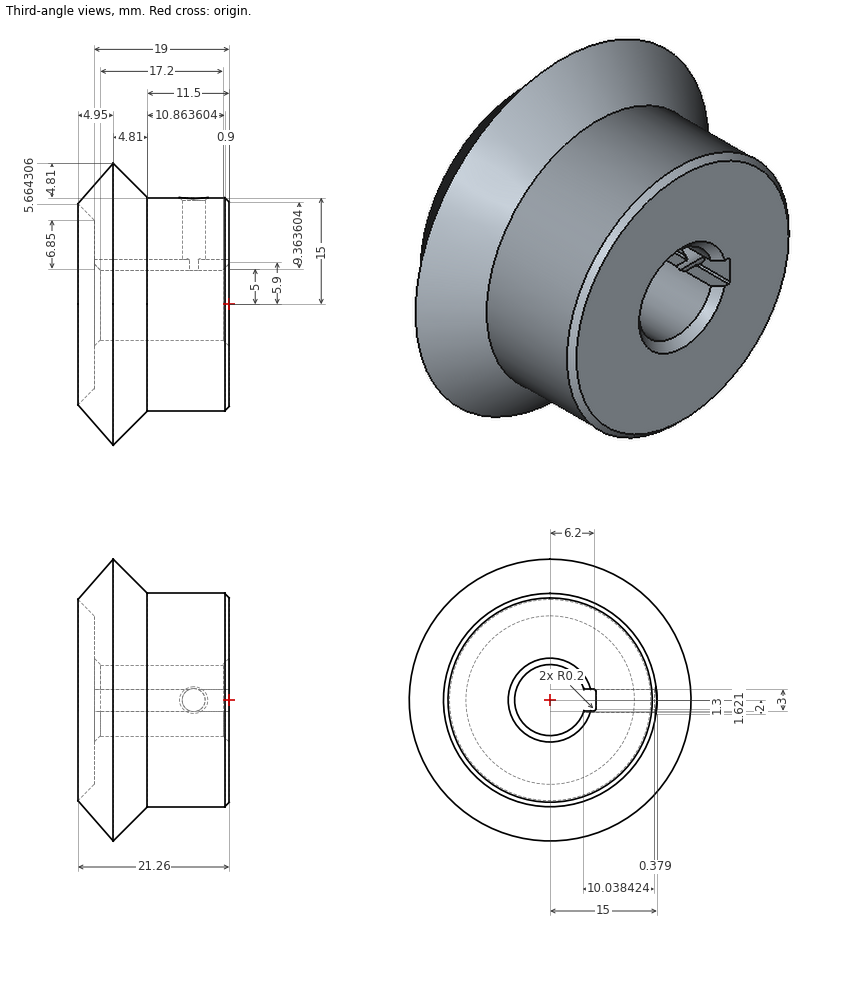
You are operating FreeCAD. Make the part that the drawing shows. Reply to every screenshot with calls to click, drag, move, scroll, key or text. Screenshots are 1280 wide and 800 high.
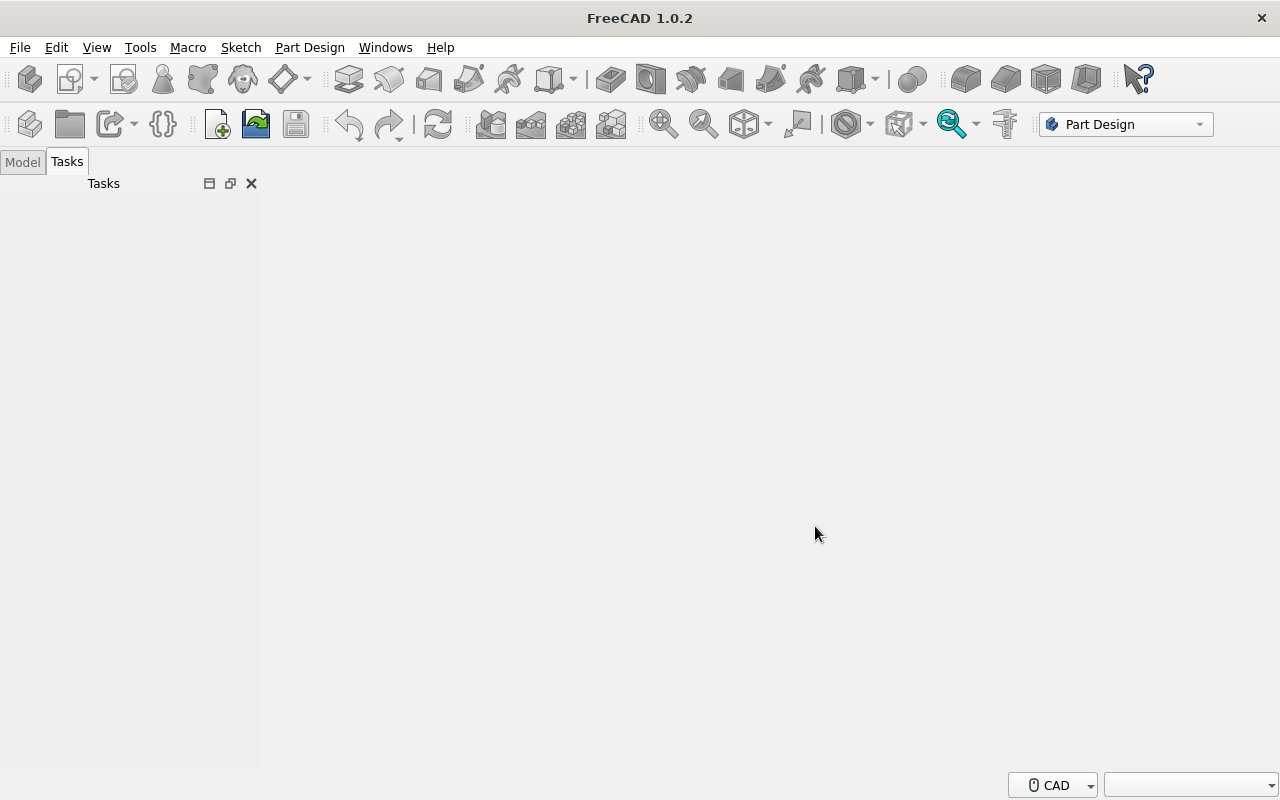
key(ctrl+n)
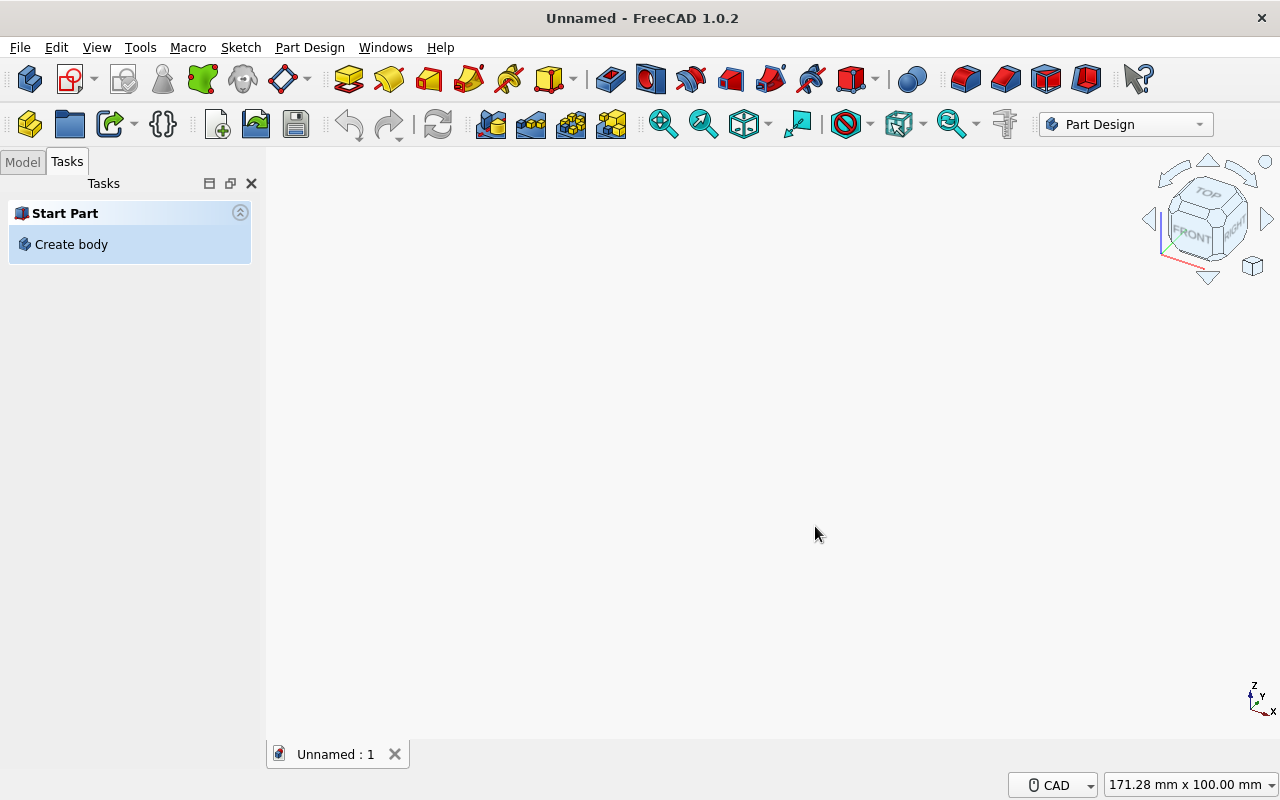
click(70, 80)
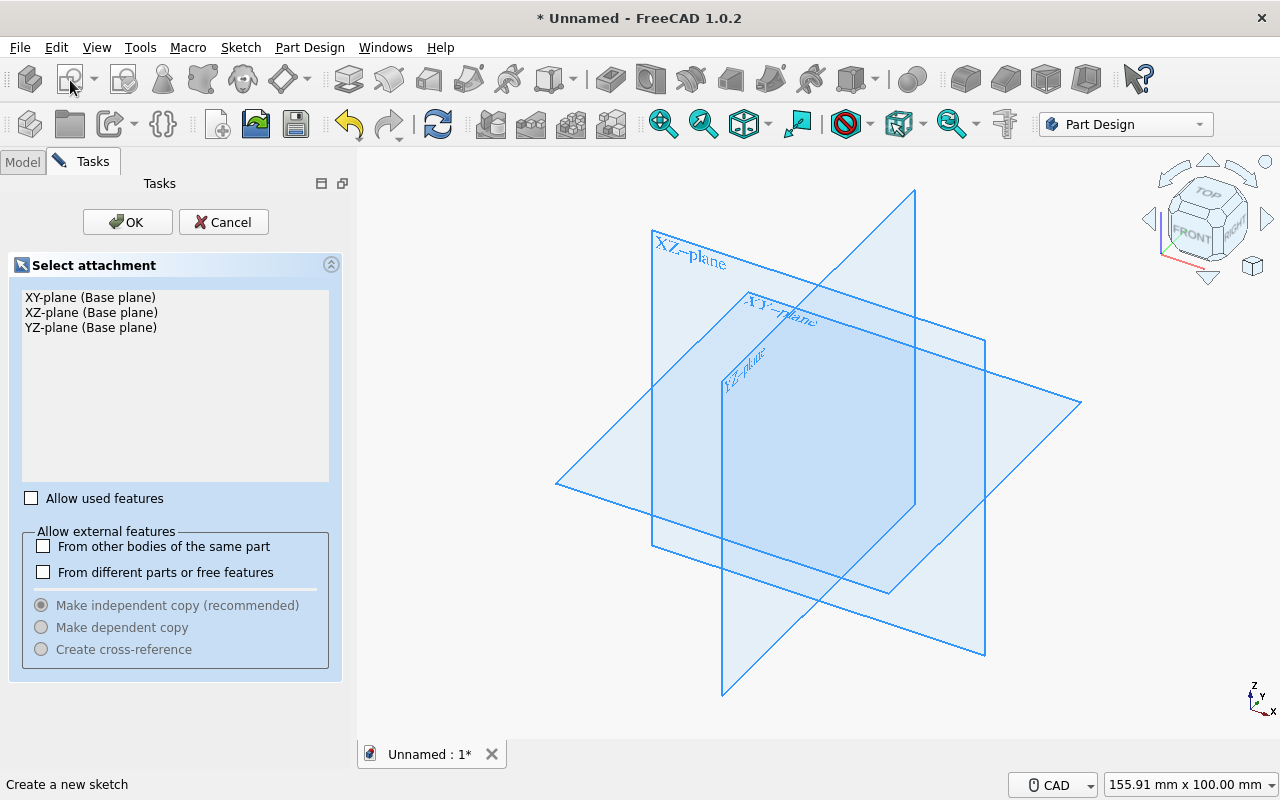
click(82, 298)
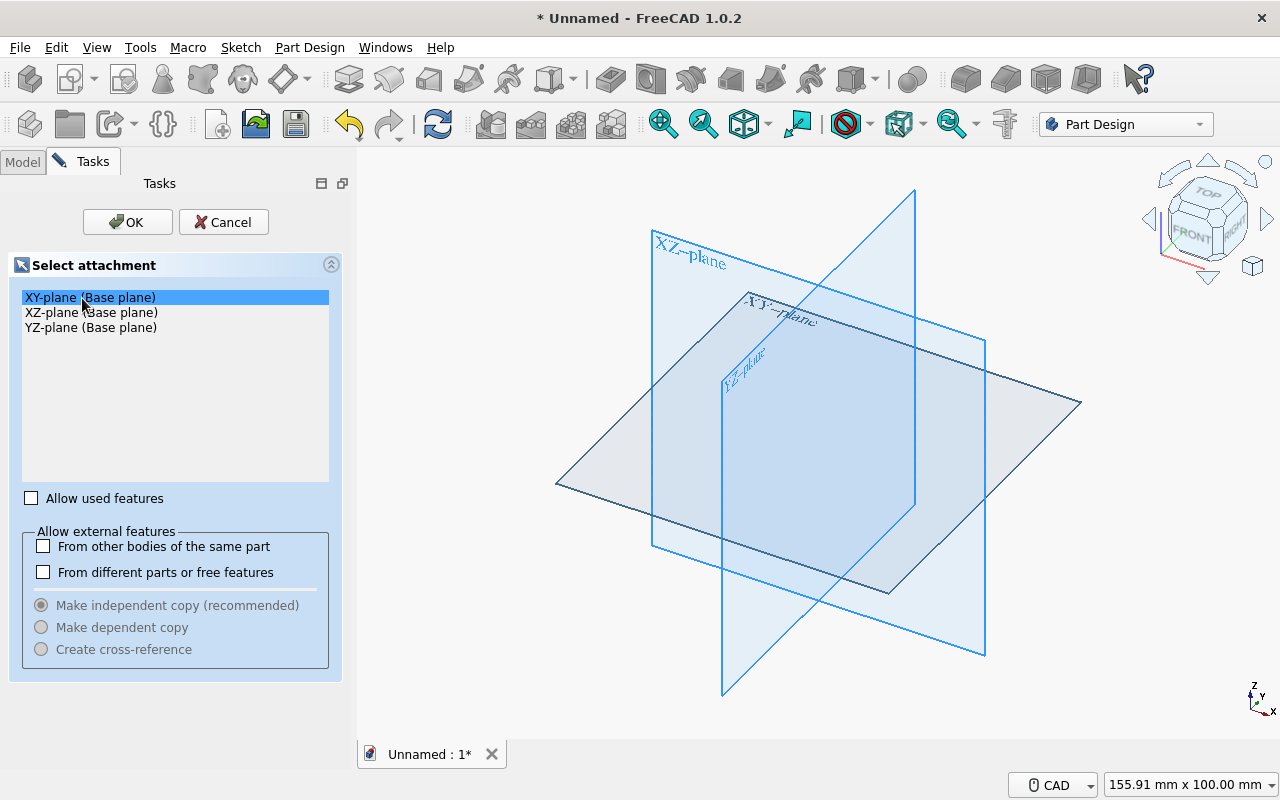
click(128, 222)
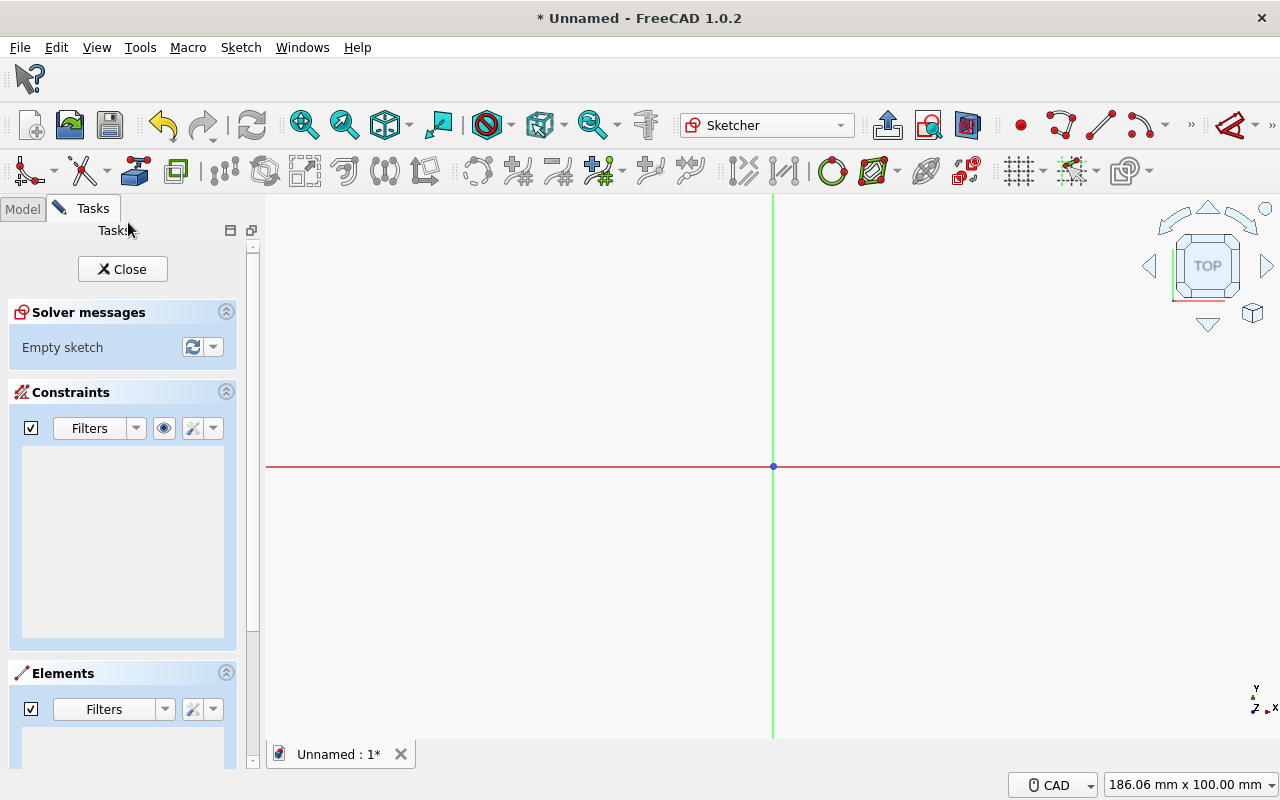
scroll(720, 389, up, 6)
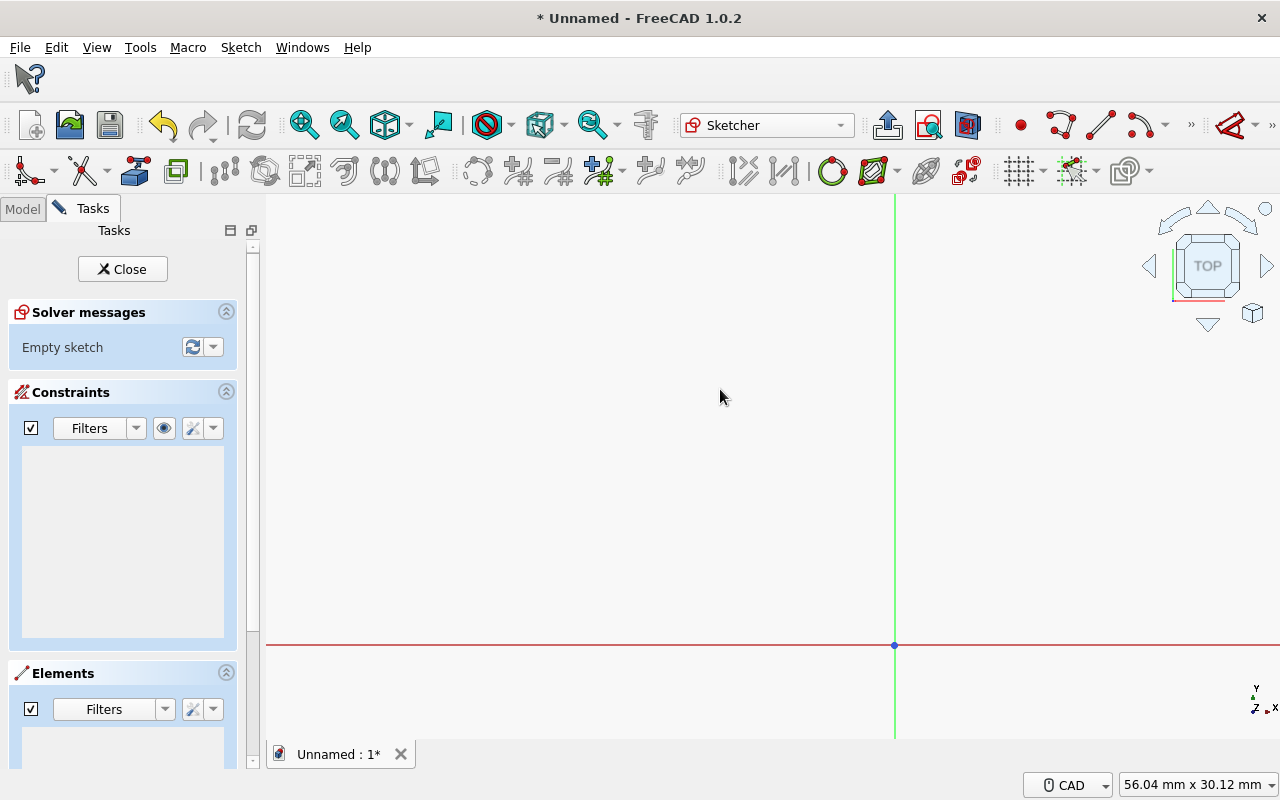
click(1062, 126)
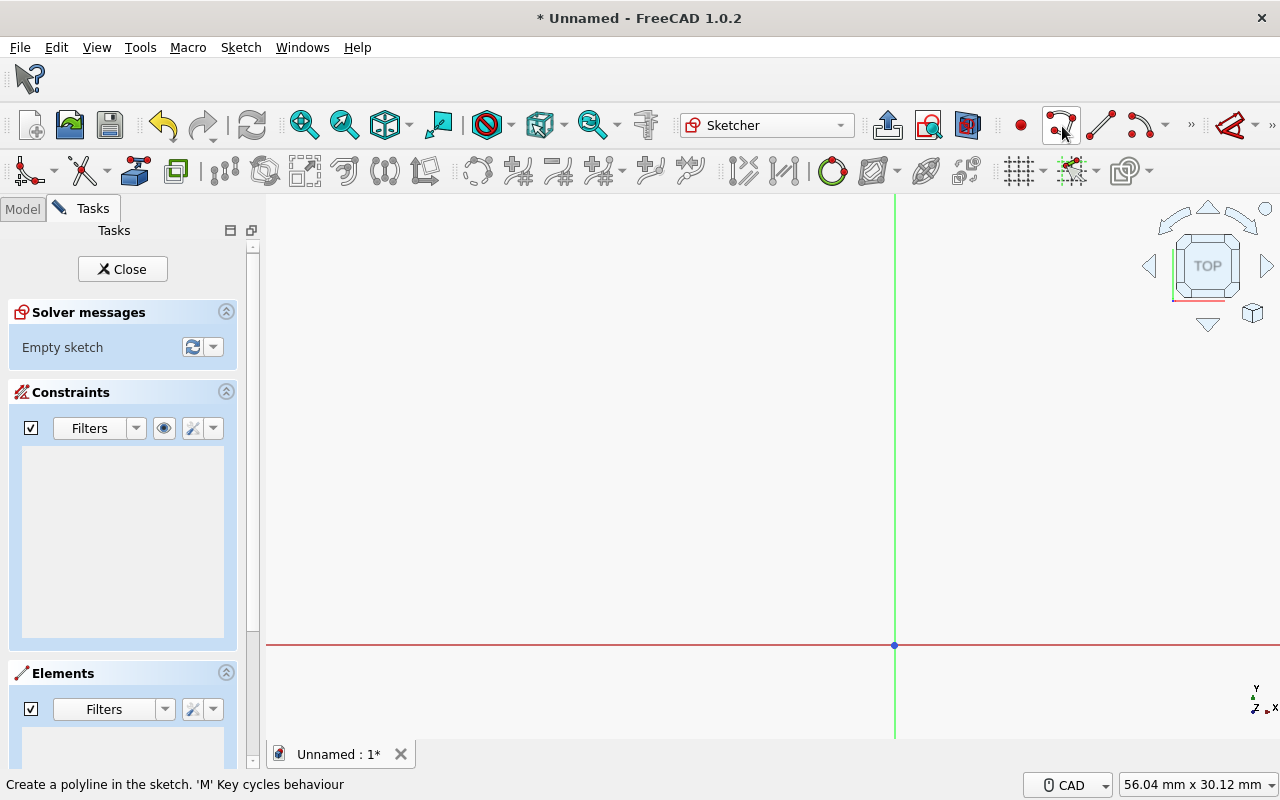
click(895, 555)
click(886, 386)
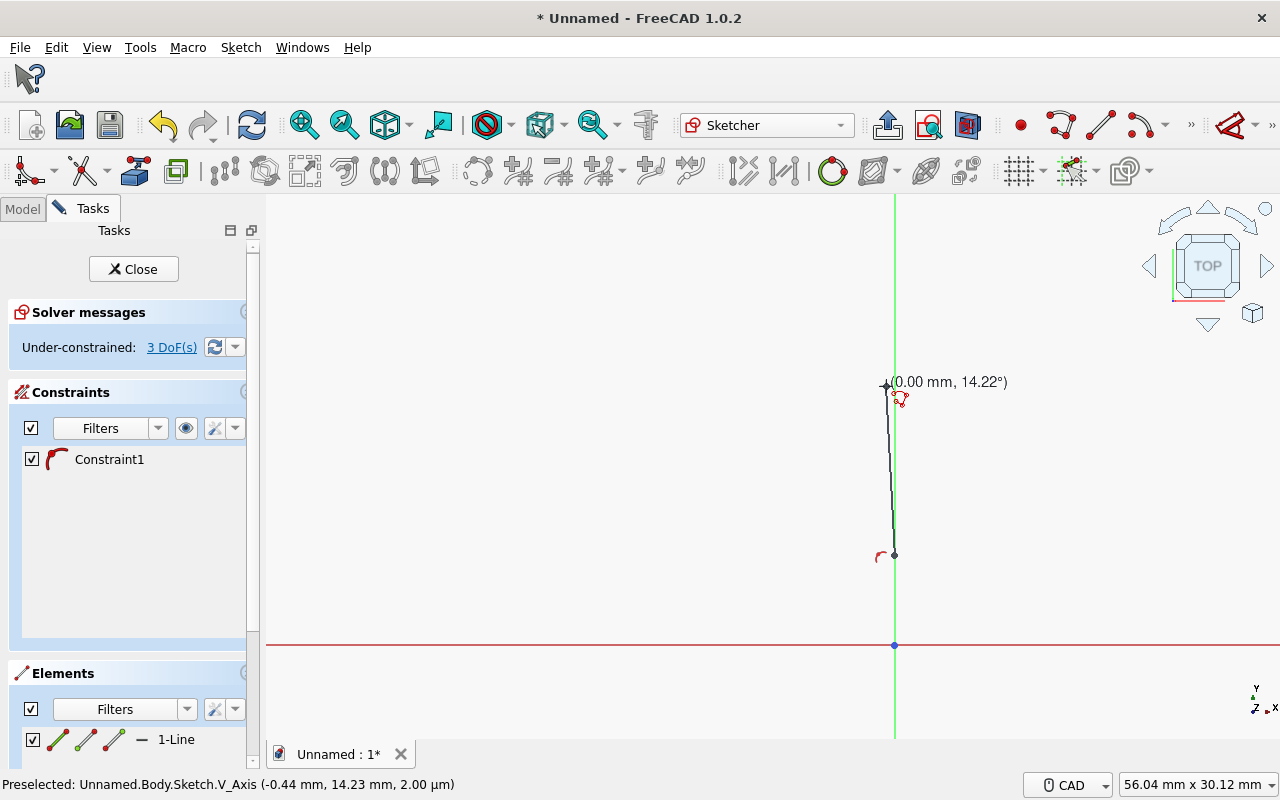
scroll(883, 374, up, 2)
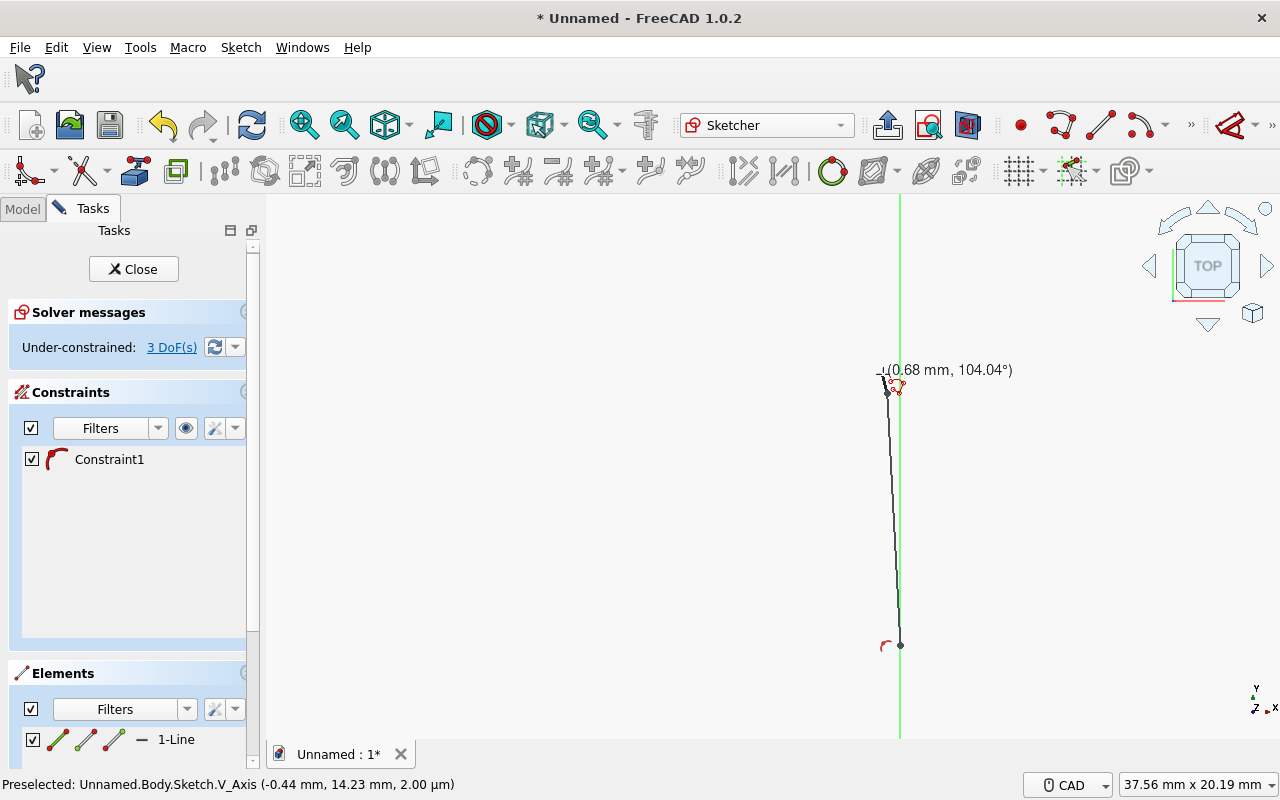
click(883, 374)
click(590, 374)
click(460, 244)
click(327, 397)
click(388, 459)
click(388, 644)
click(900, 645)
key(Escape)
key(Escape)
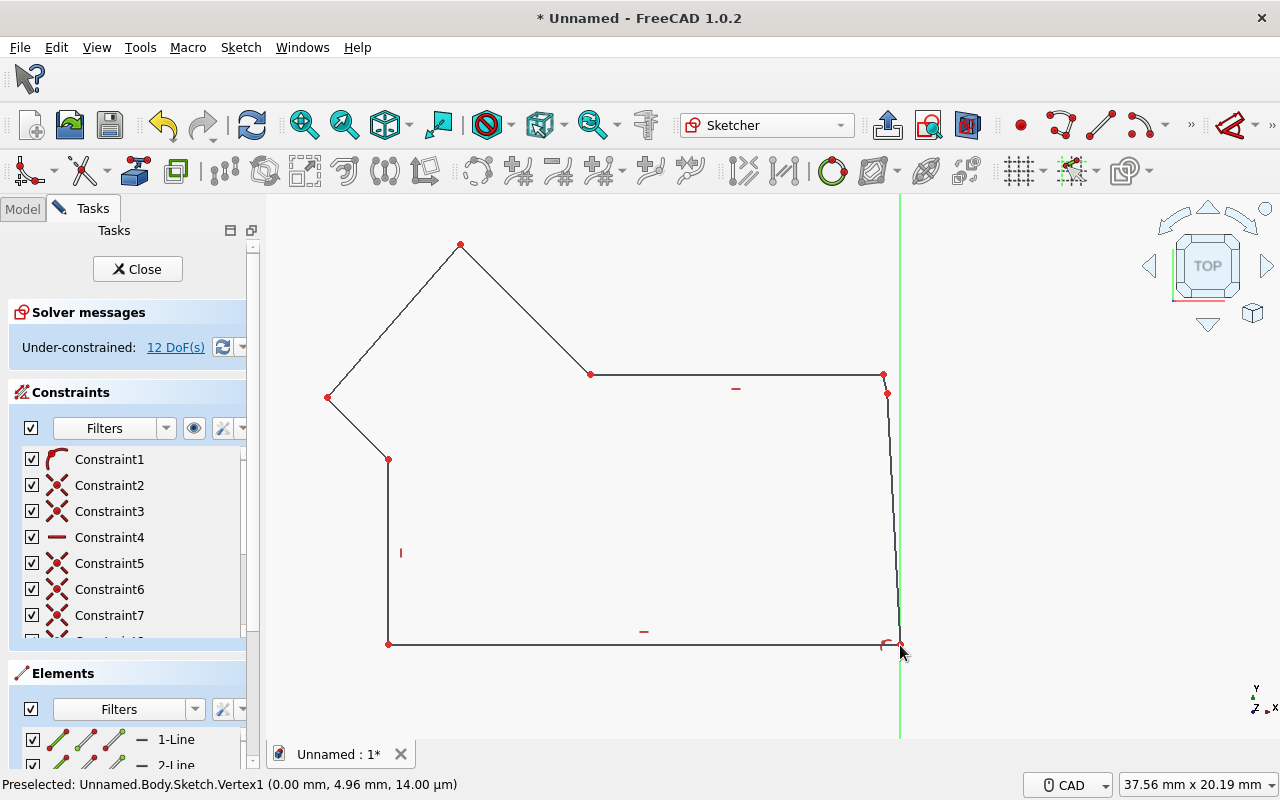
click(896, 569)